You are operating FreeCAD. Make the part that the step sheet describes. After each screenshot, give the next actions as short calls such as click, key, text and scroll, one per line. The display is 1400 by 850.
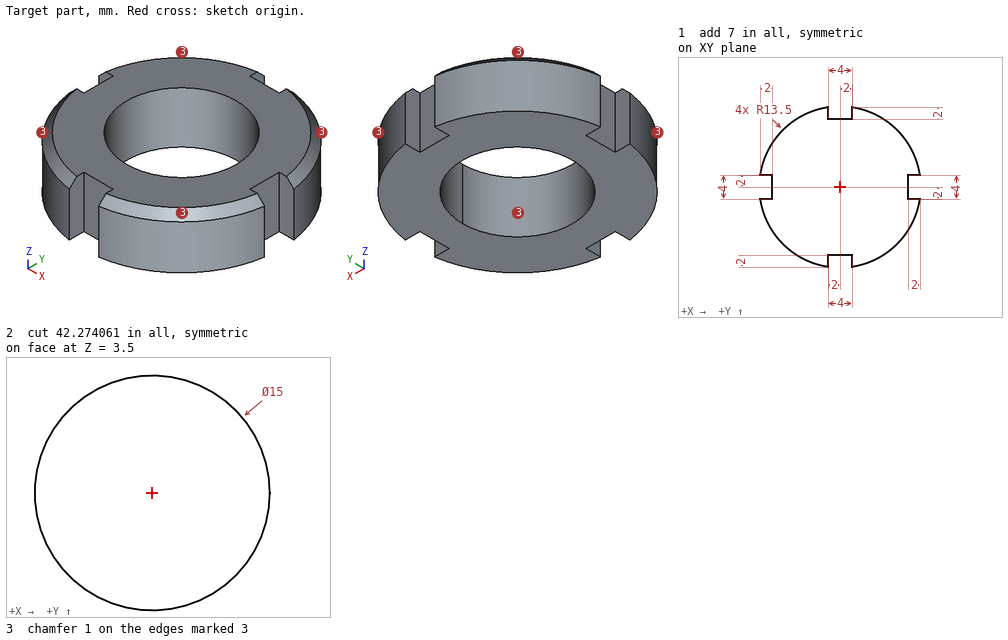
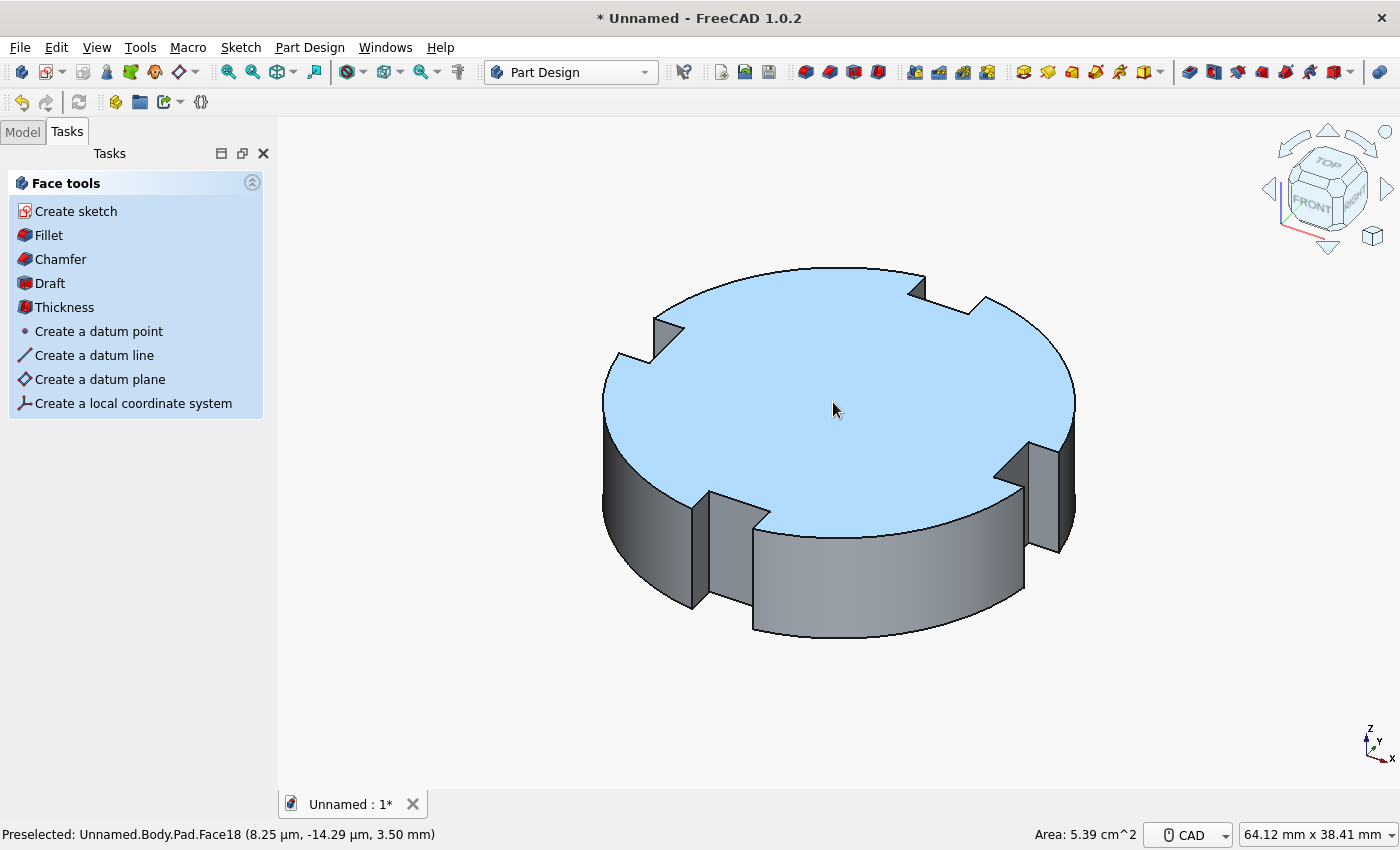
click(46, 72)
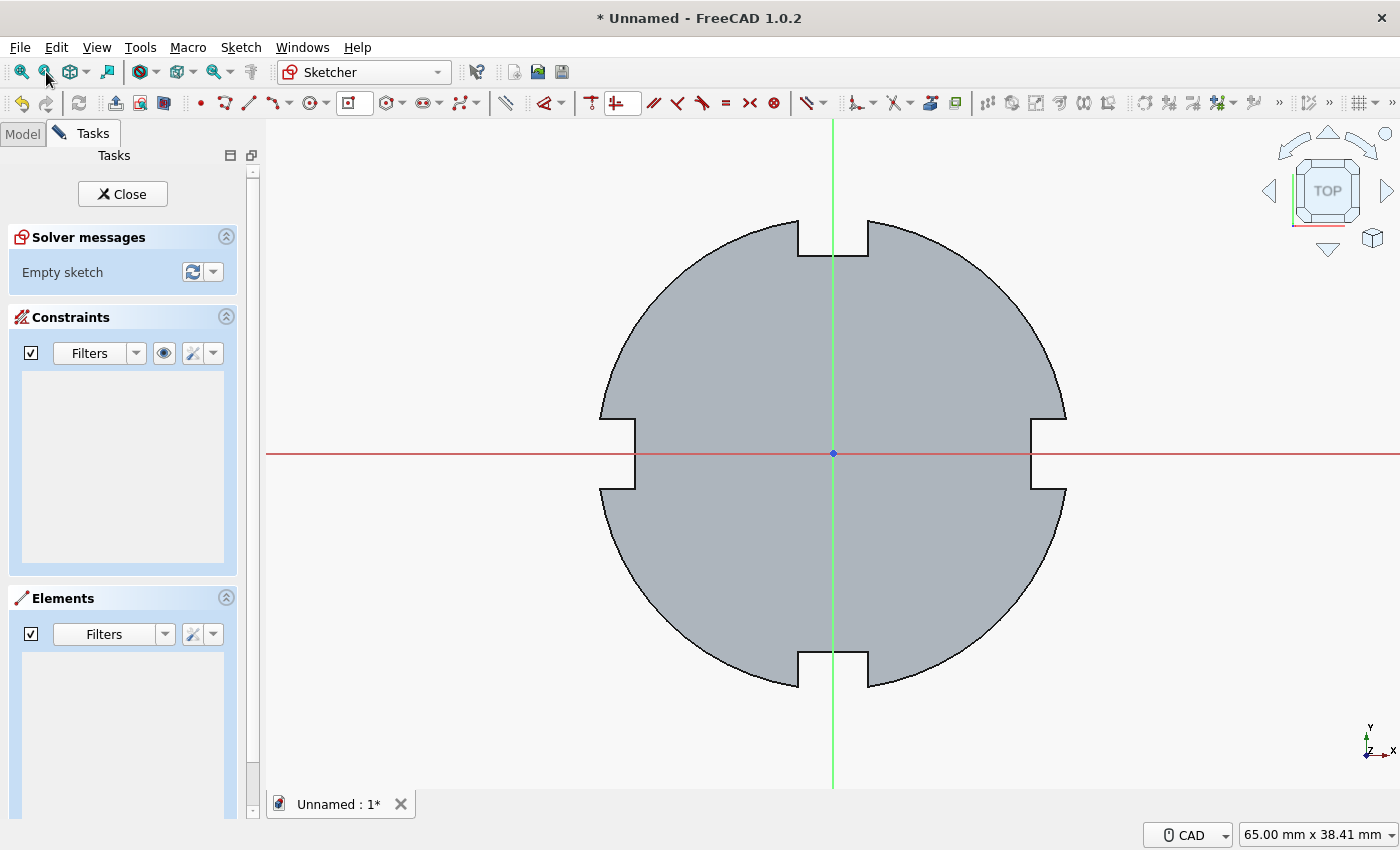
scroll(916, 454, up, 3)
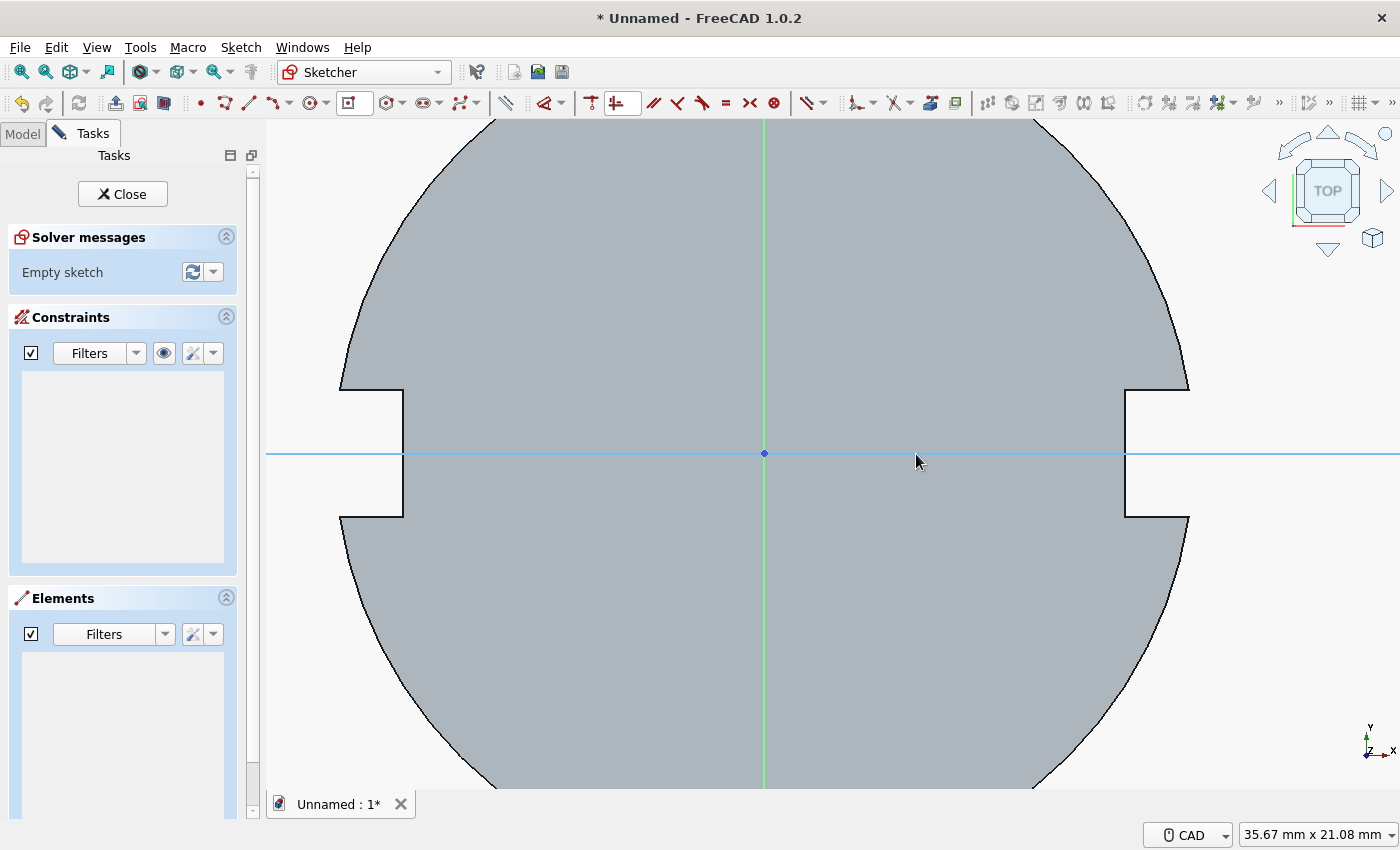
key(g)
key(c)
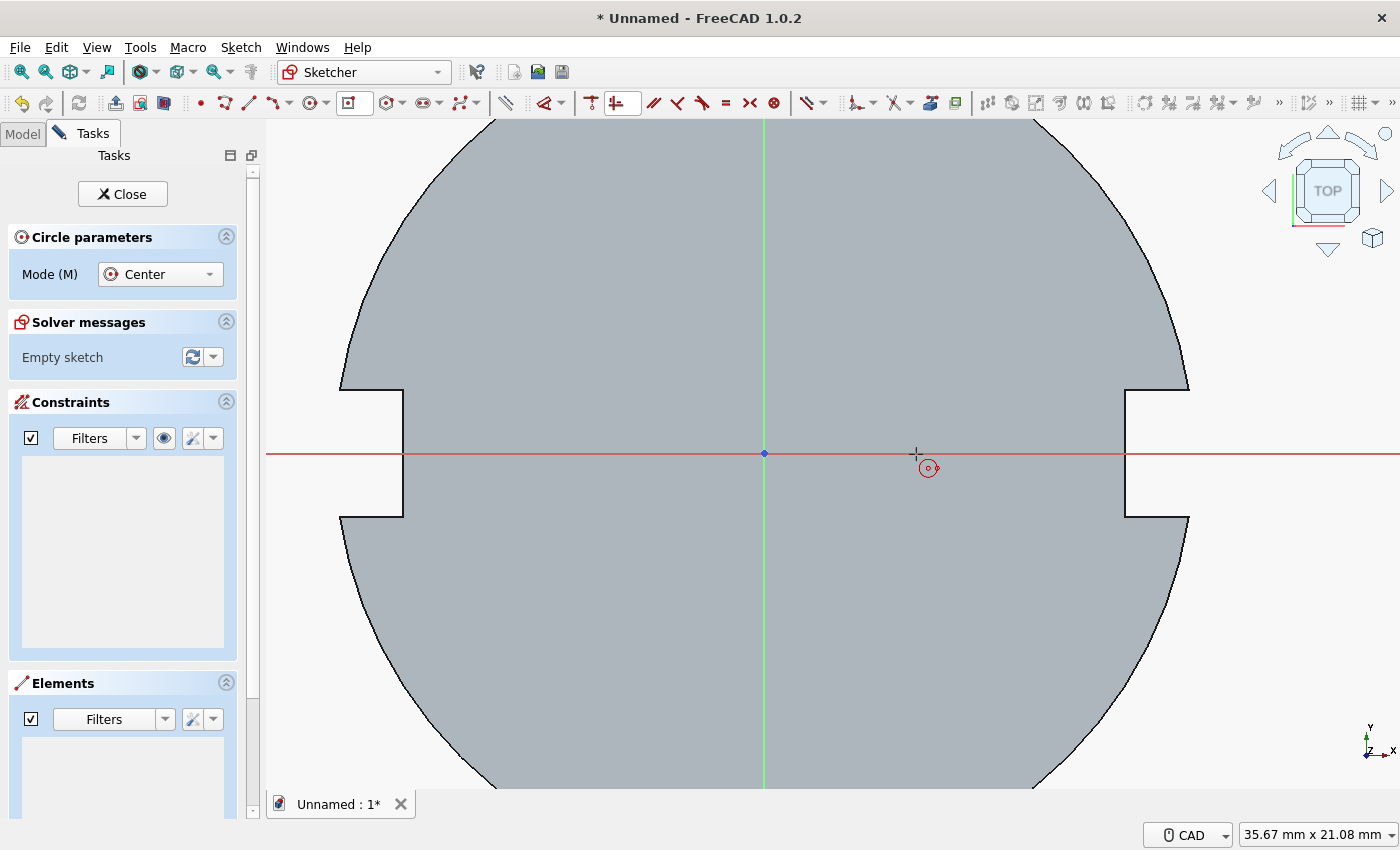
click(764, 454)
click(933, 285)
key(Escape)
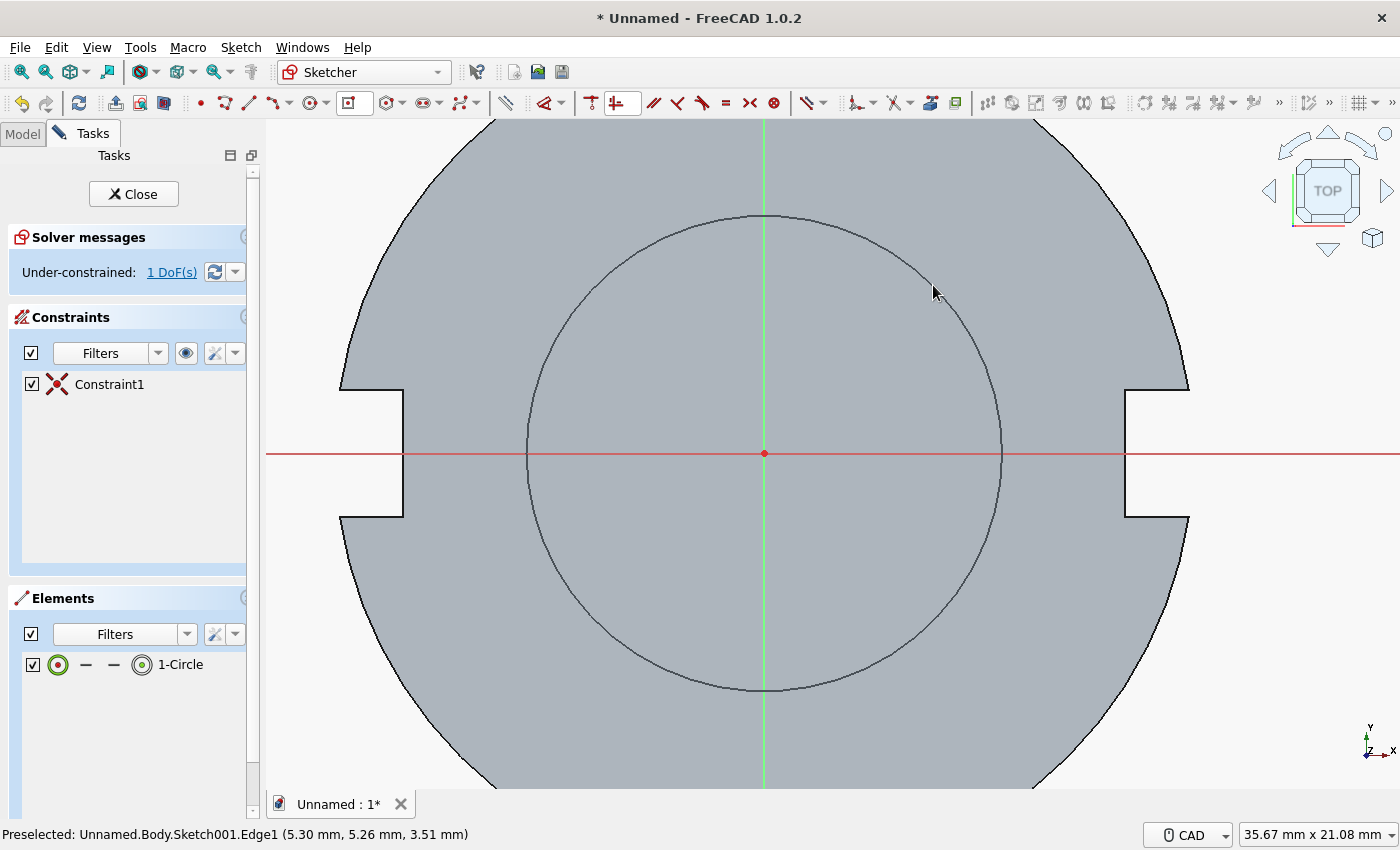
key(d)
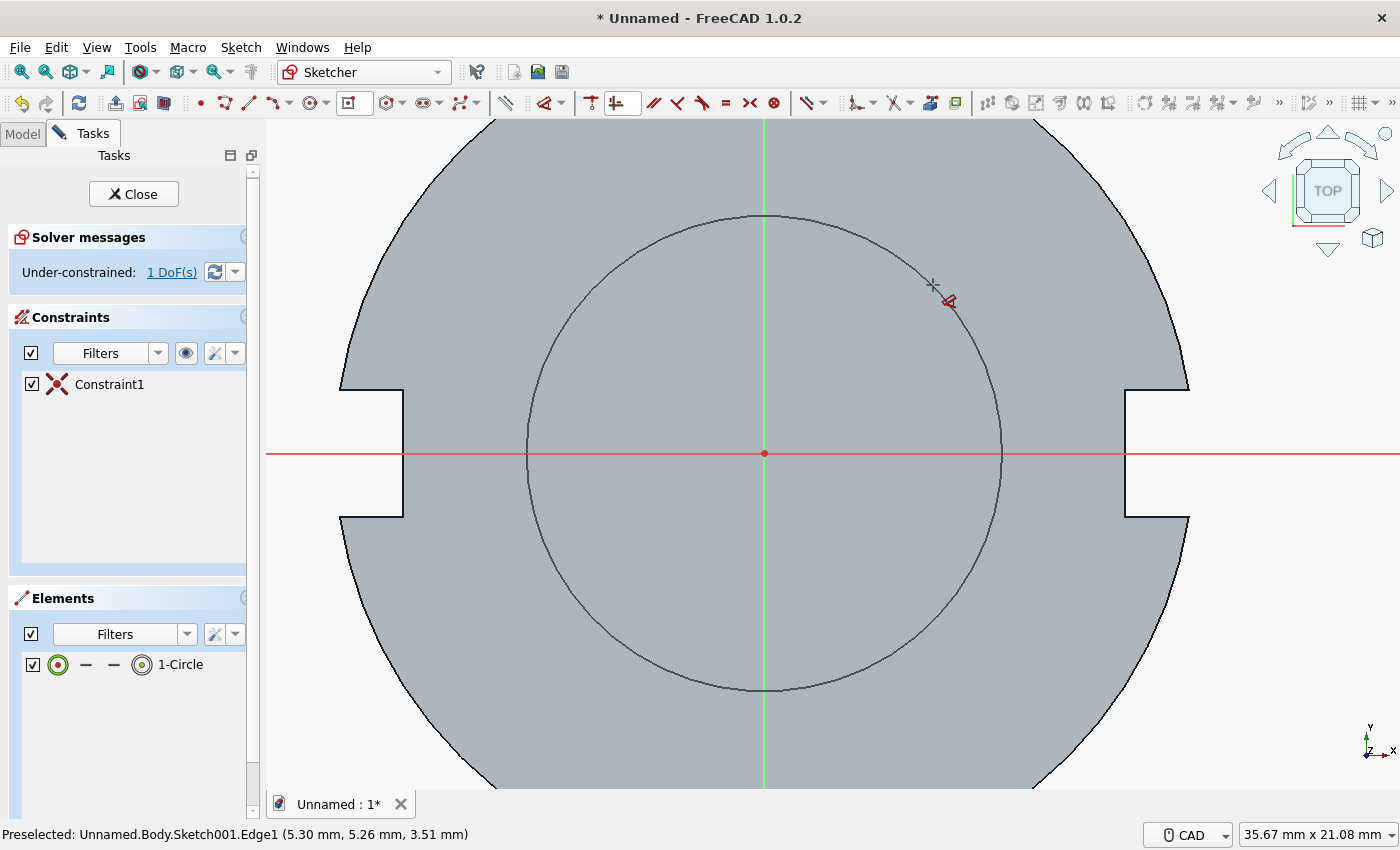
click(932, 285)
click(955, 262)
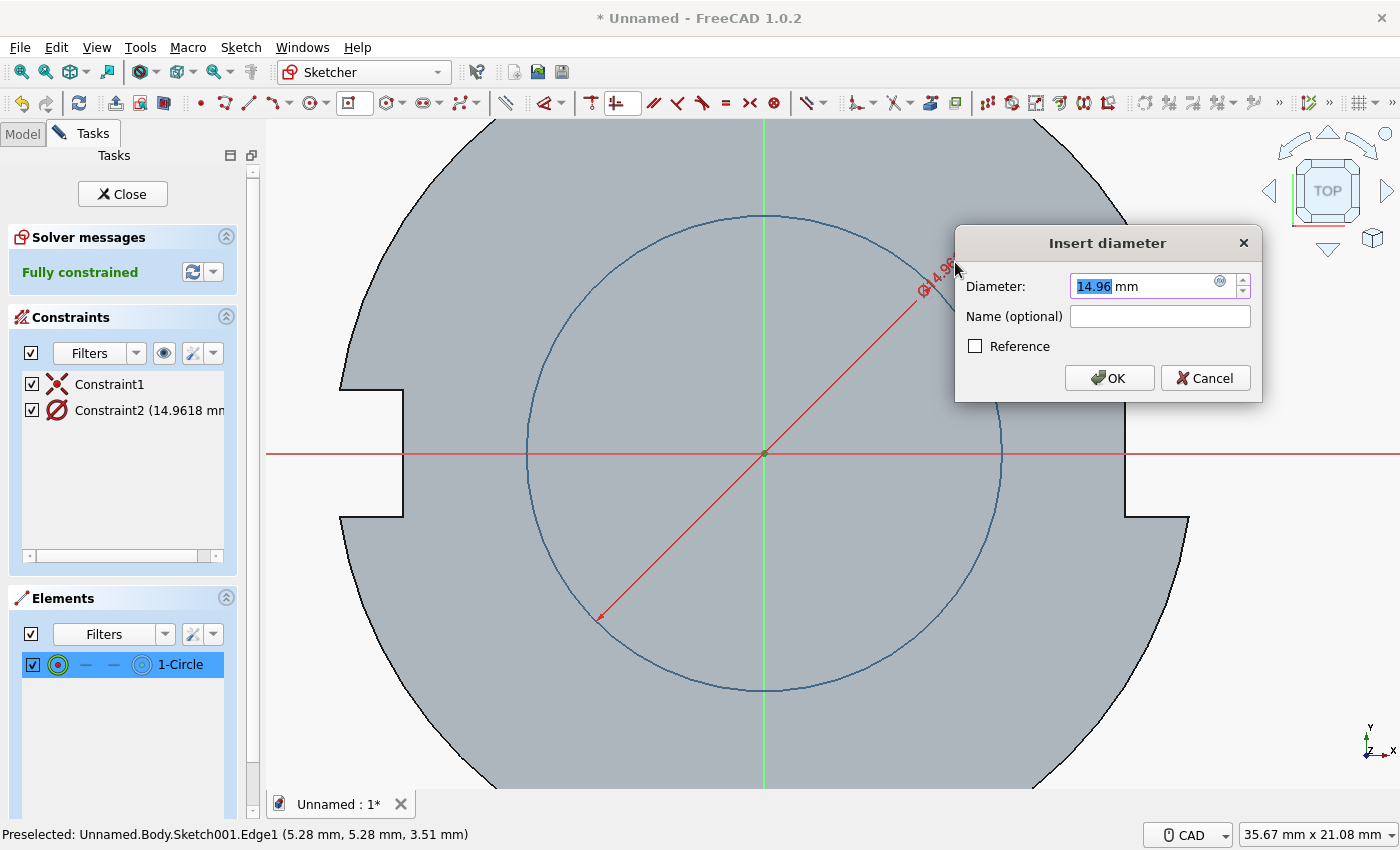
text(15)
key(Return)
key(Escape)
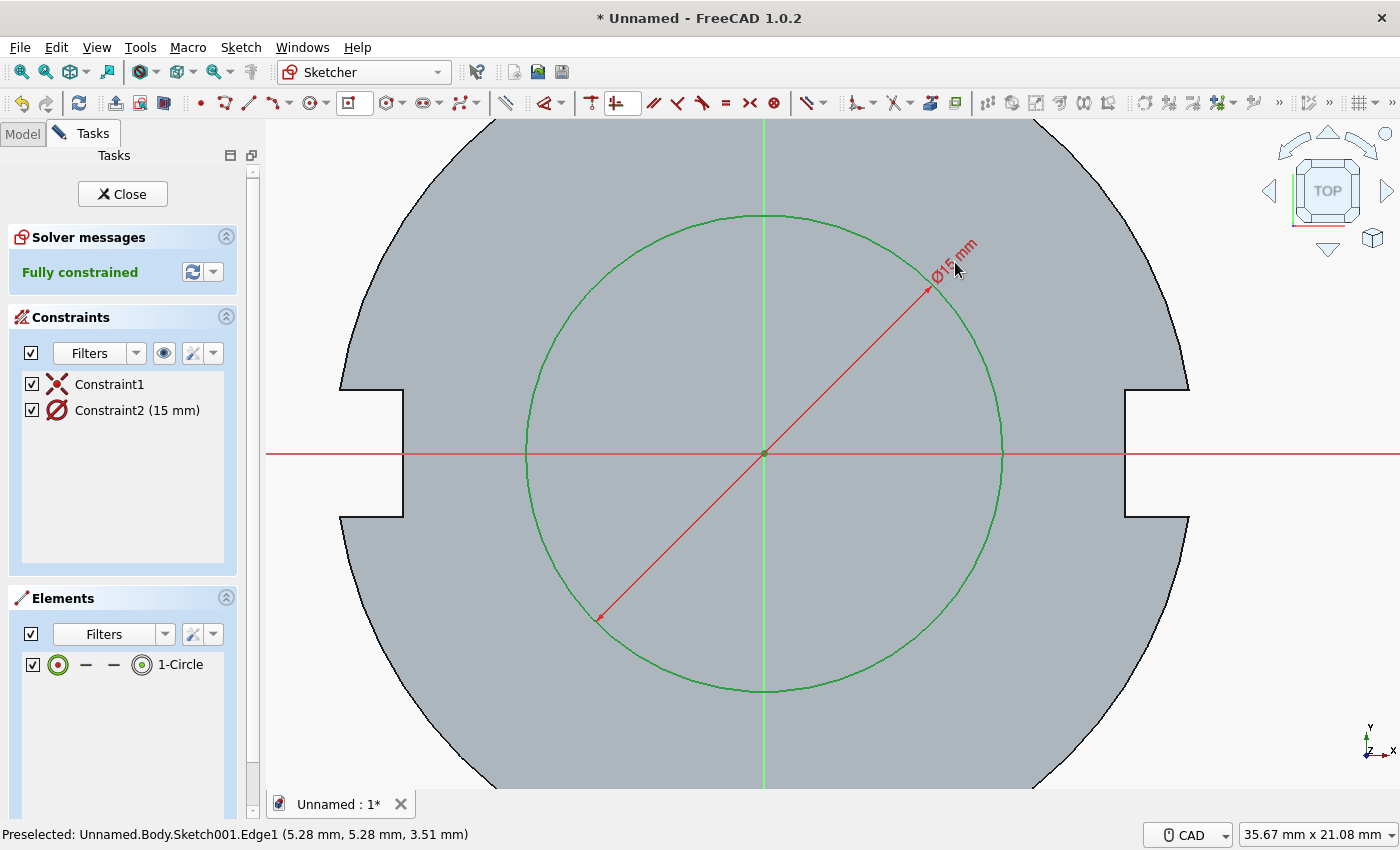
click(123, 194)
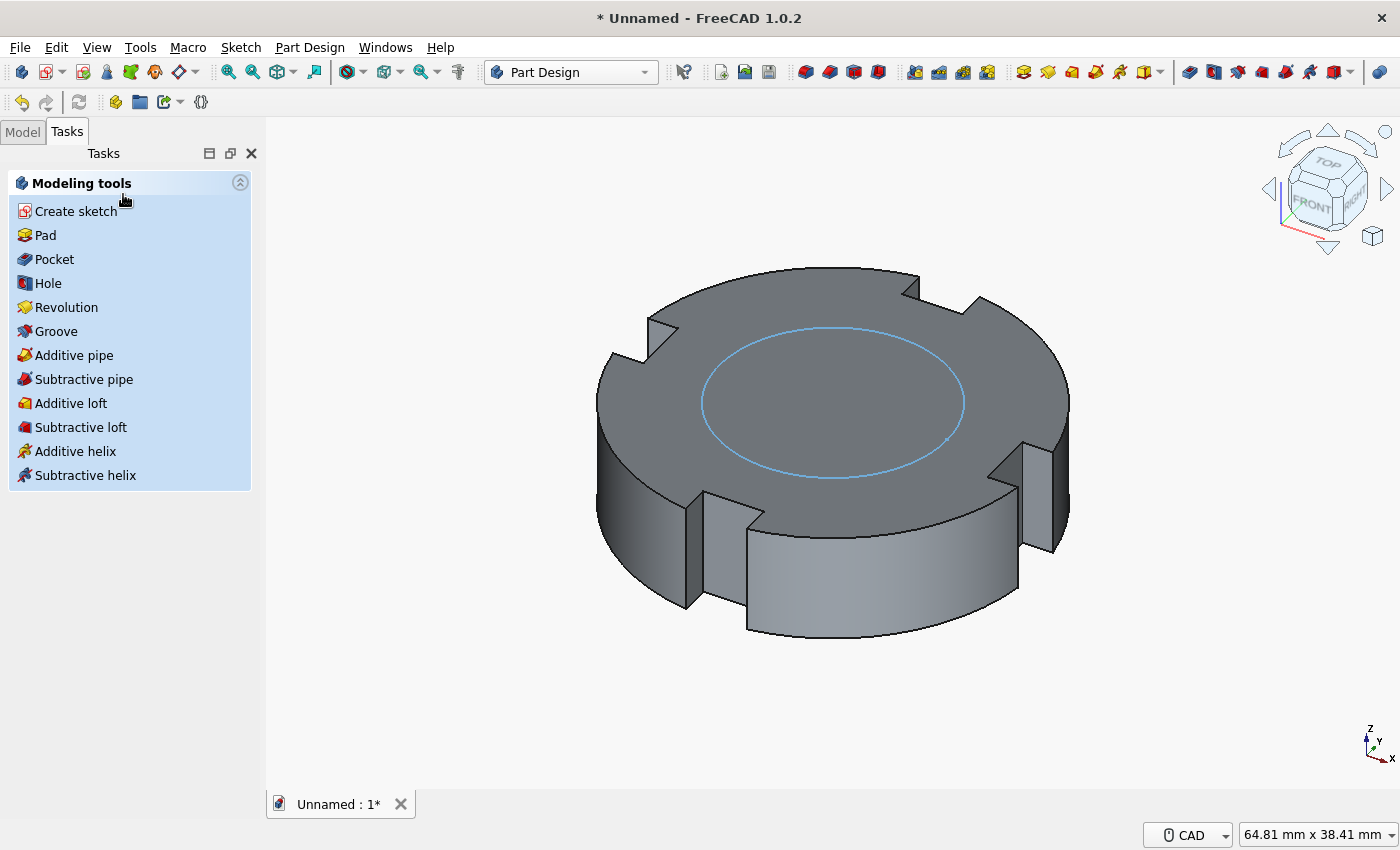
click(1190, 72)